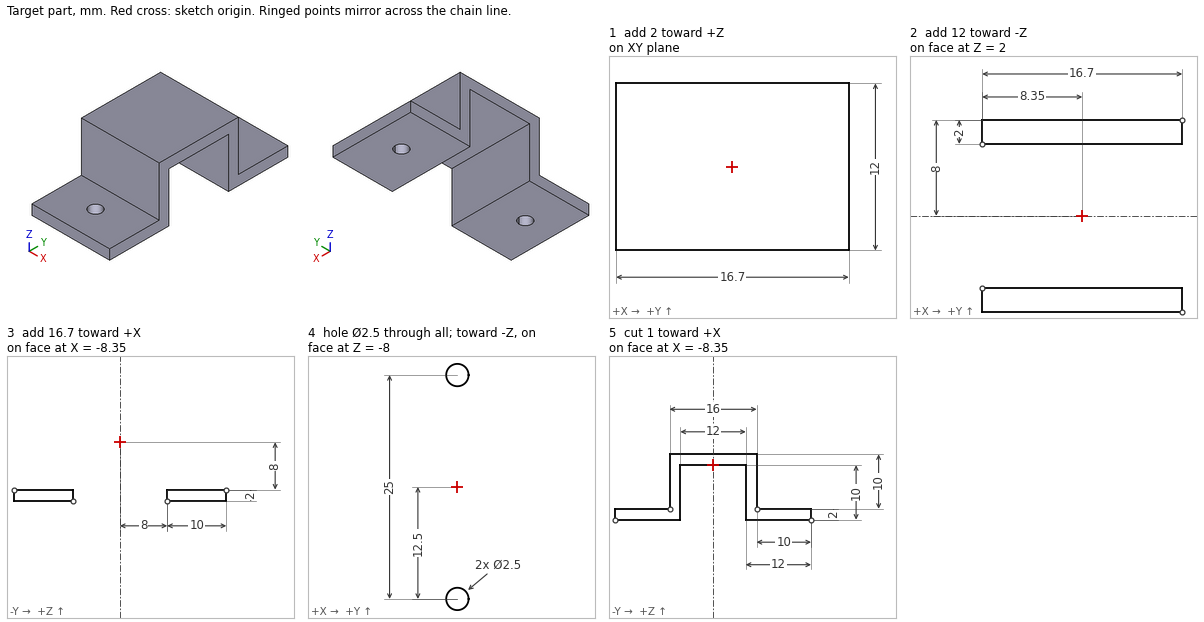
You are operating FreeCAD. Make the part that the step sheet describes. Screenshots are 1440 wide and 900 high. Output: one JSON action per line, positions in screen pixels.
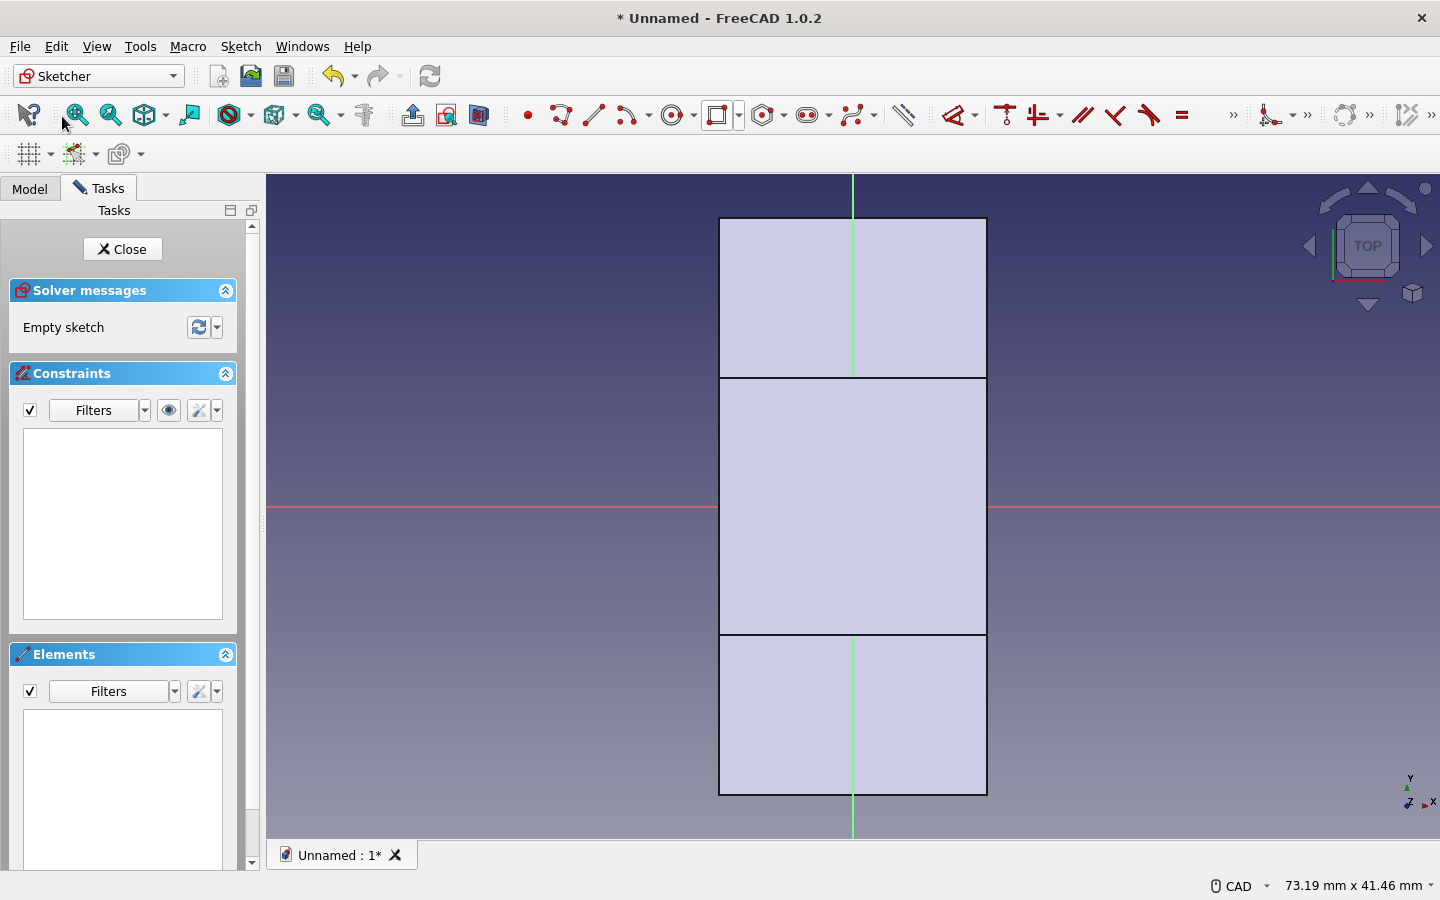
{"action": "left_click", "coordinate": [479, 116]}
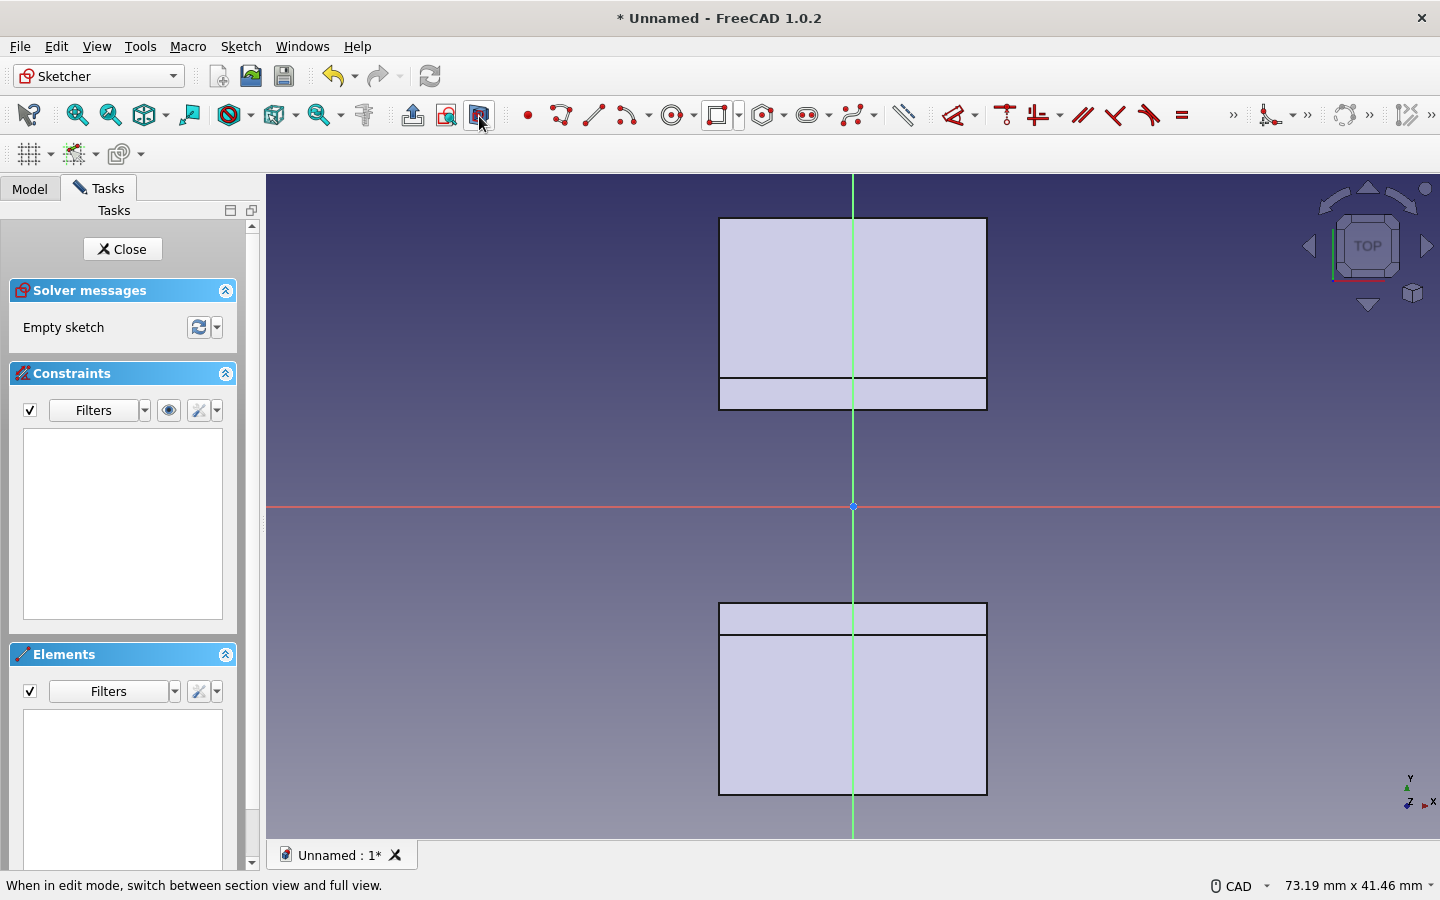
{"action": "left_click", "coordinate": [672, 116]}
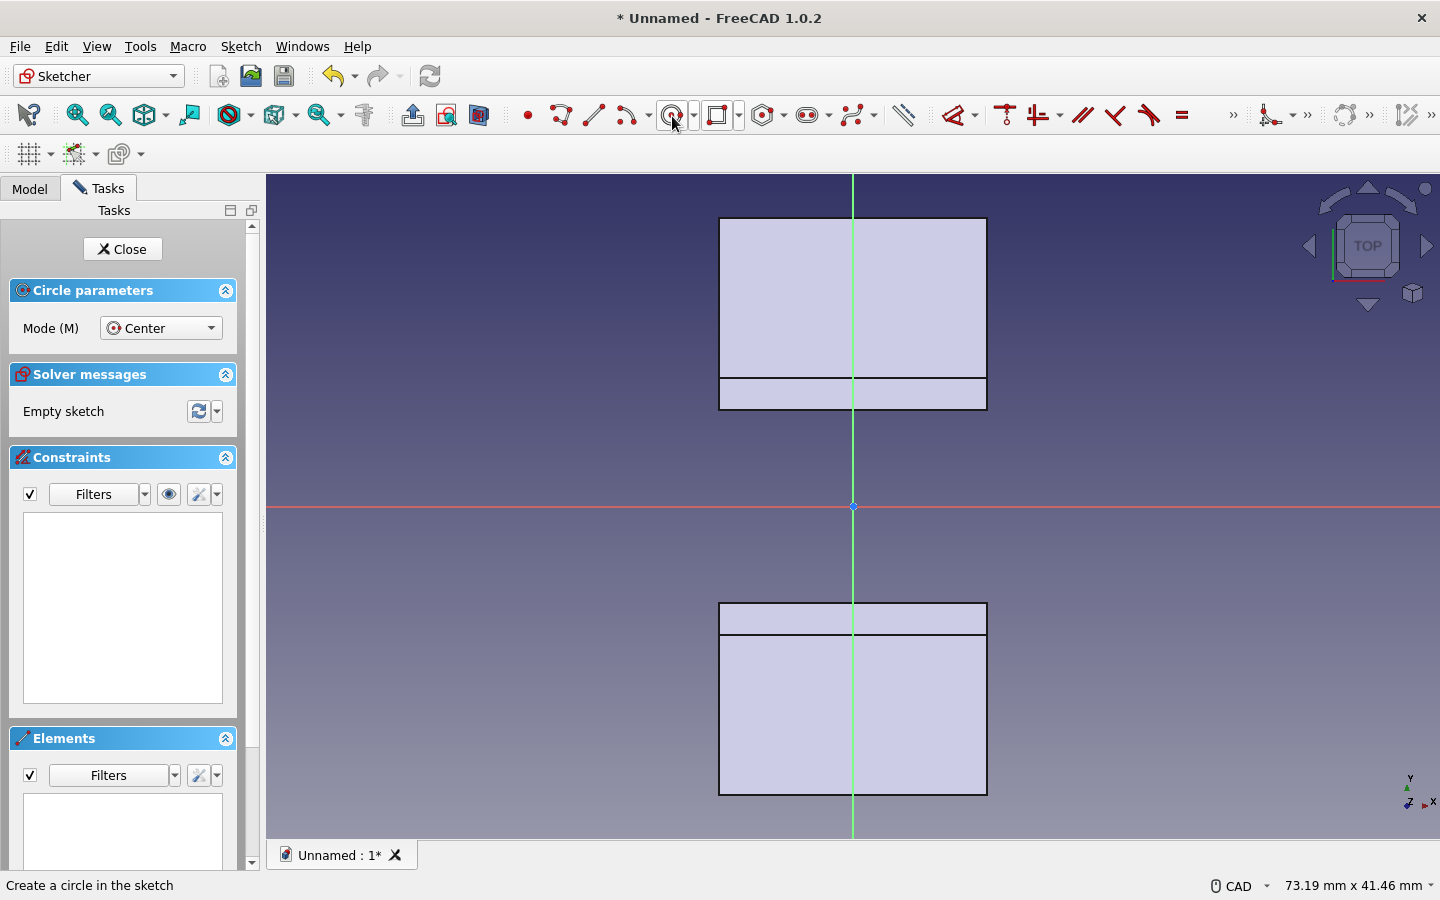
{"action": "left_click", "coordinate": [853, 707]}
{"action": "left_click", "coordinate": [867, 693]}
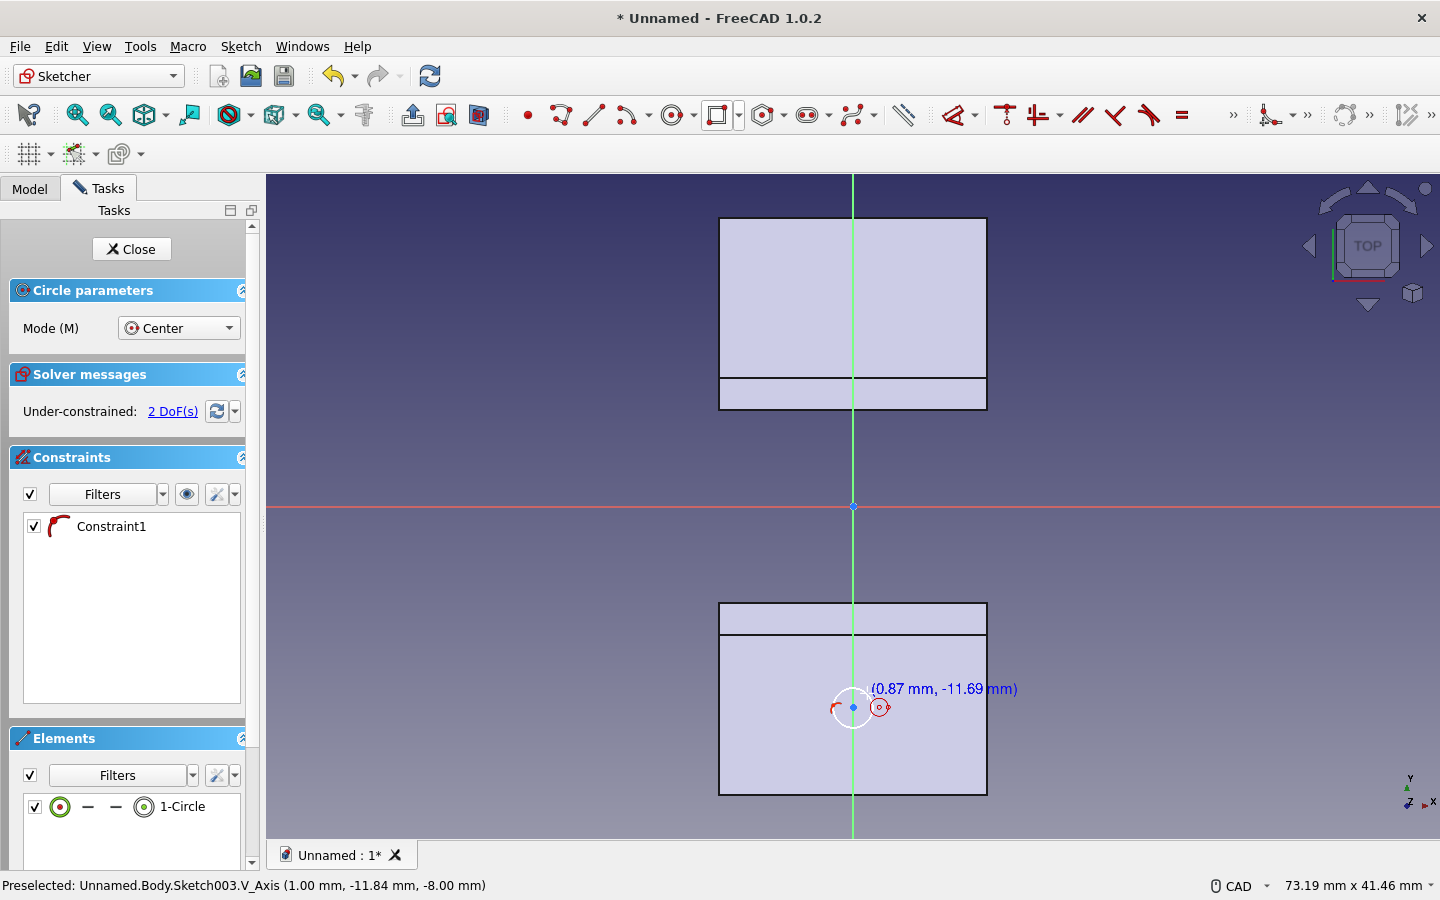
{"action": "left_click", "coordinate": [853, 306]}
{"action": "left_click", "coordinate": [867, 292]}
{"action": "key", "text": "Escape"}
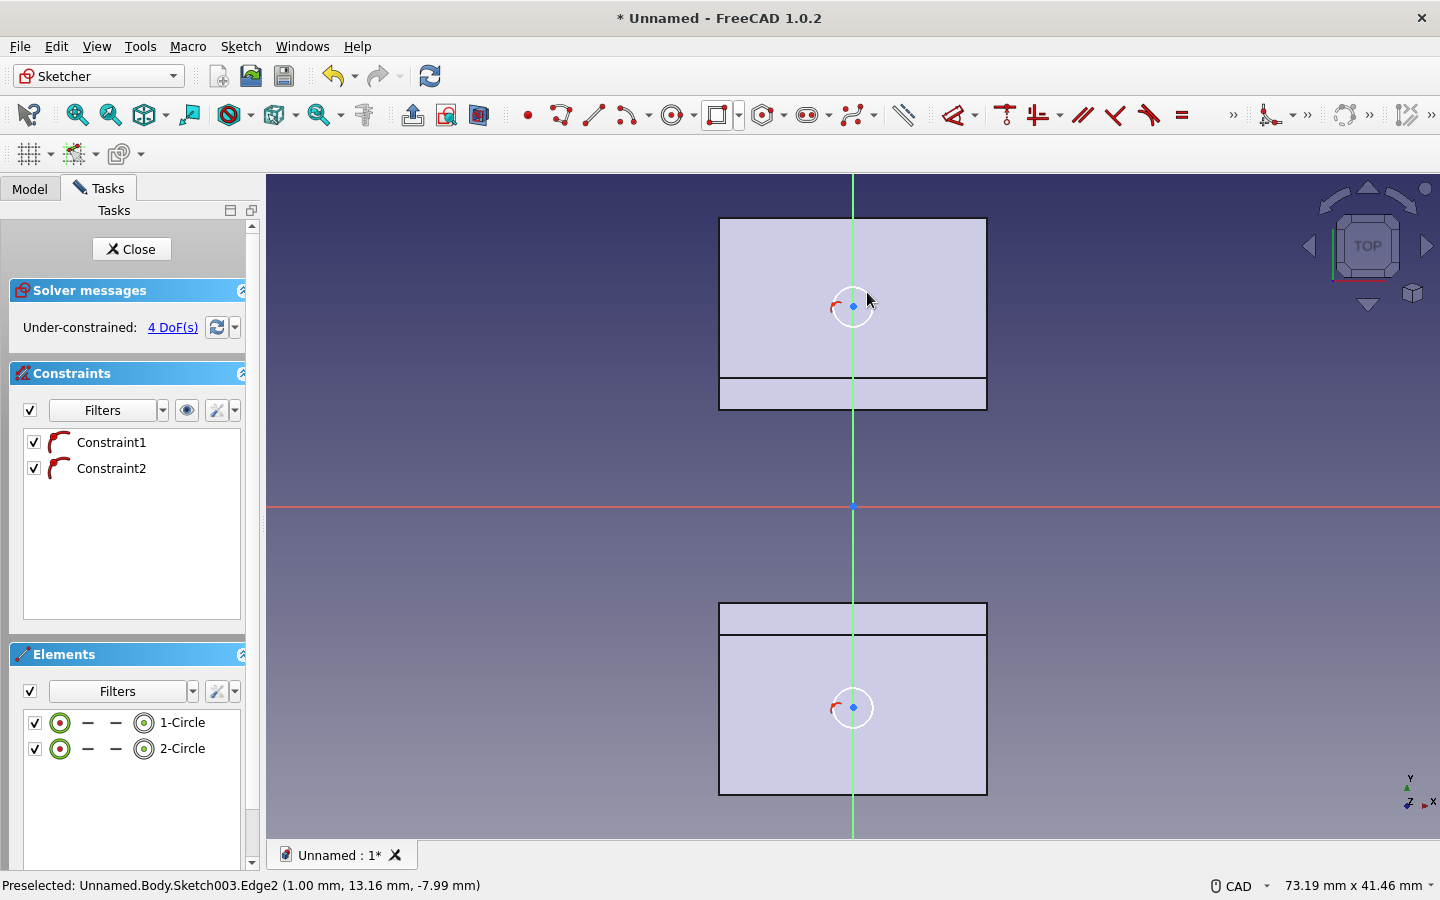
{"action": "left_click", "coordinate": [867, 694]}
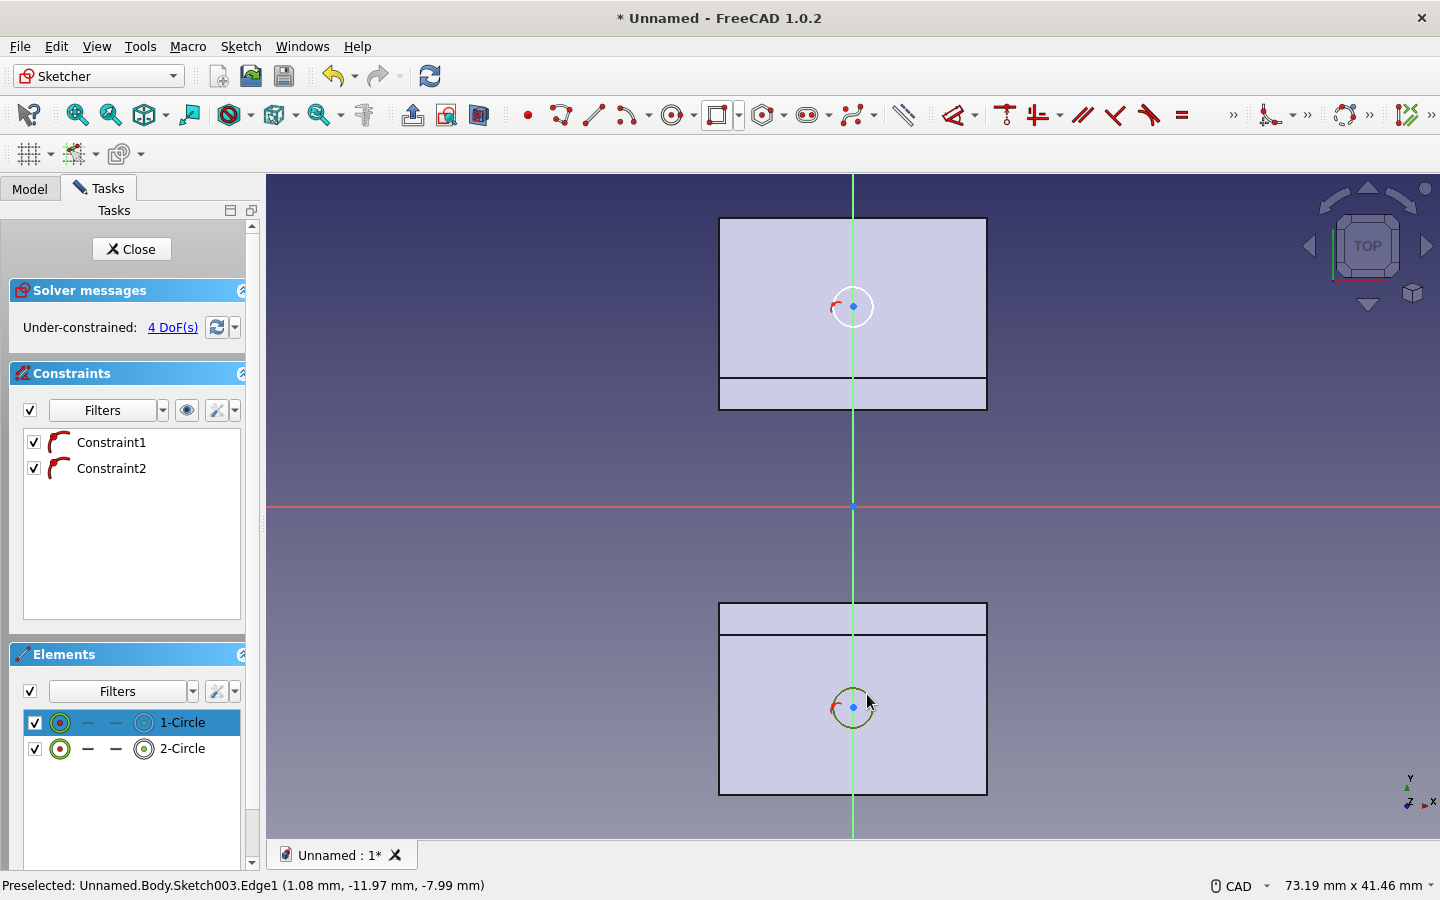
{"action": "left_click", "coordinate": [867, 293]}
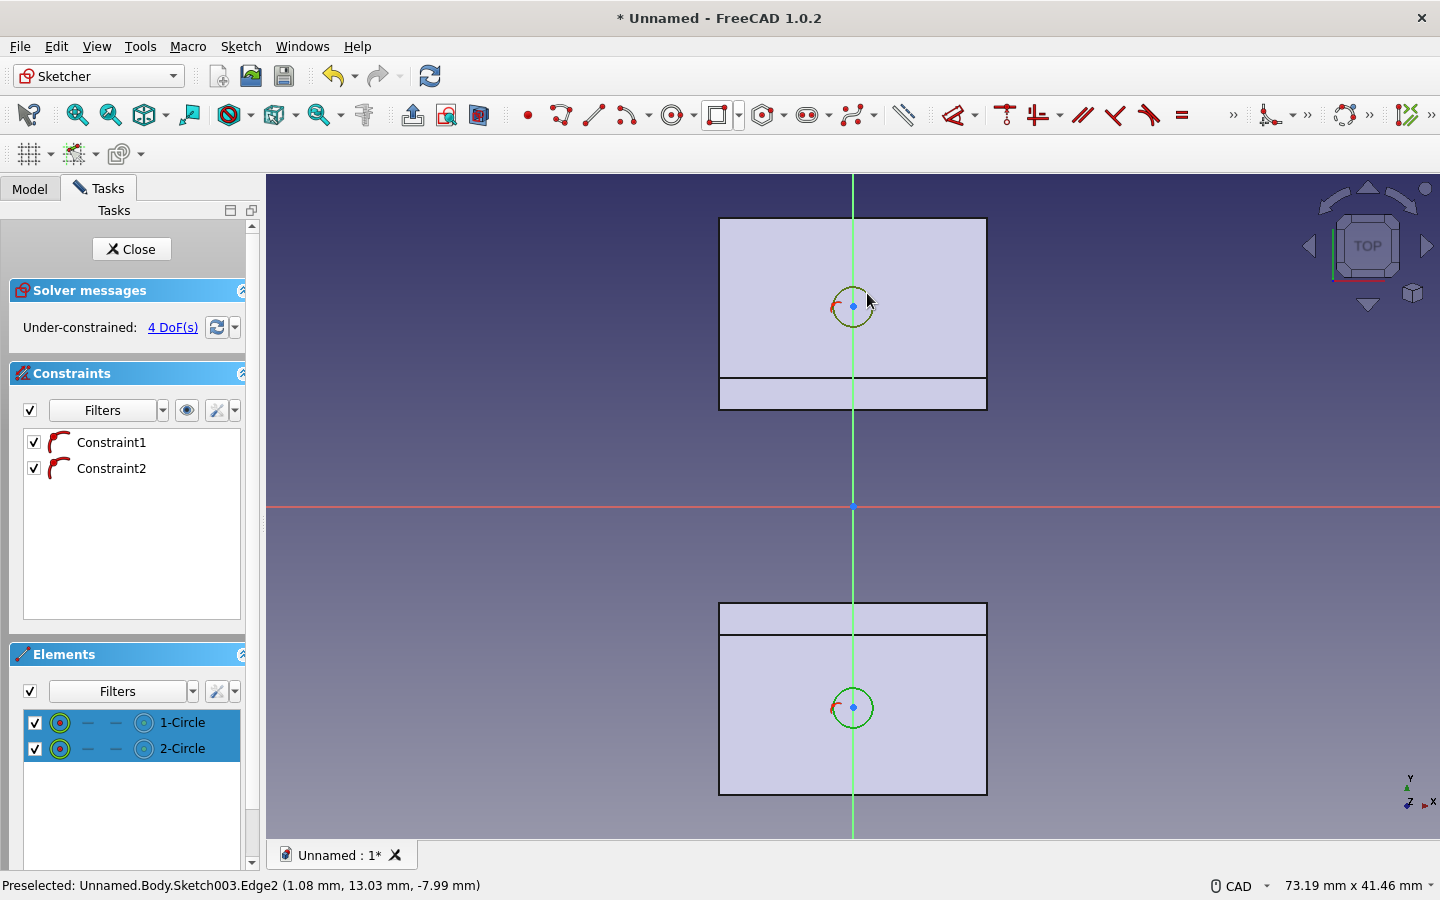
{"action": "key", "text": "e"}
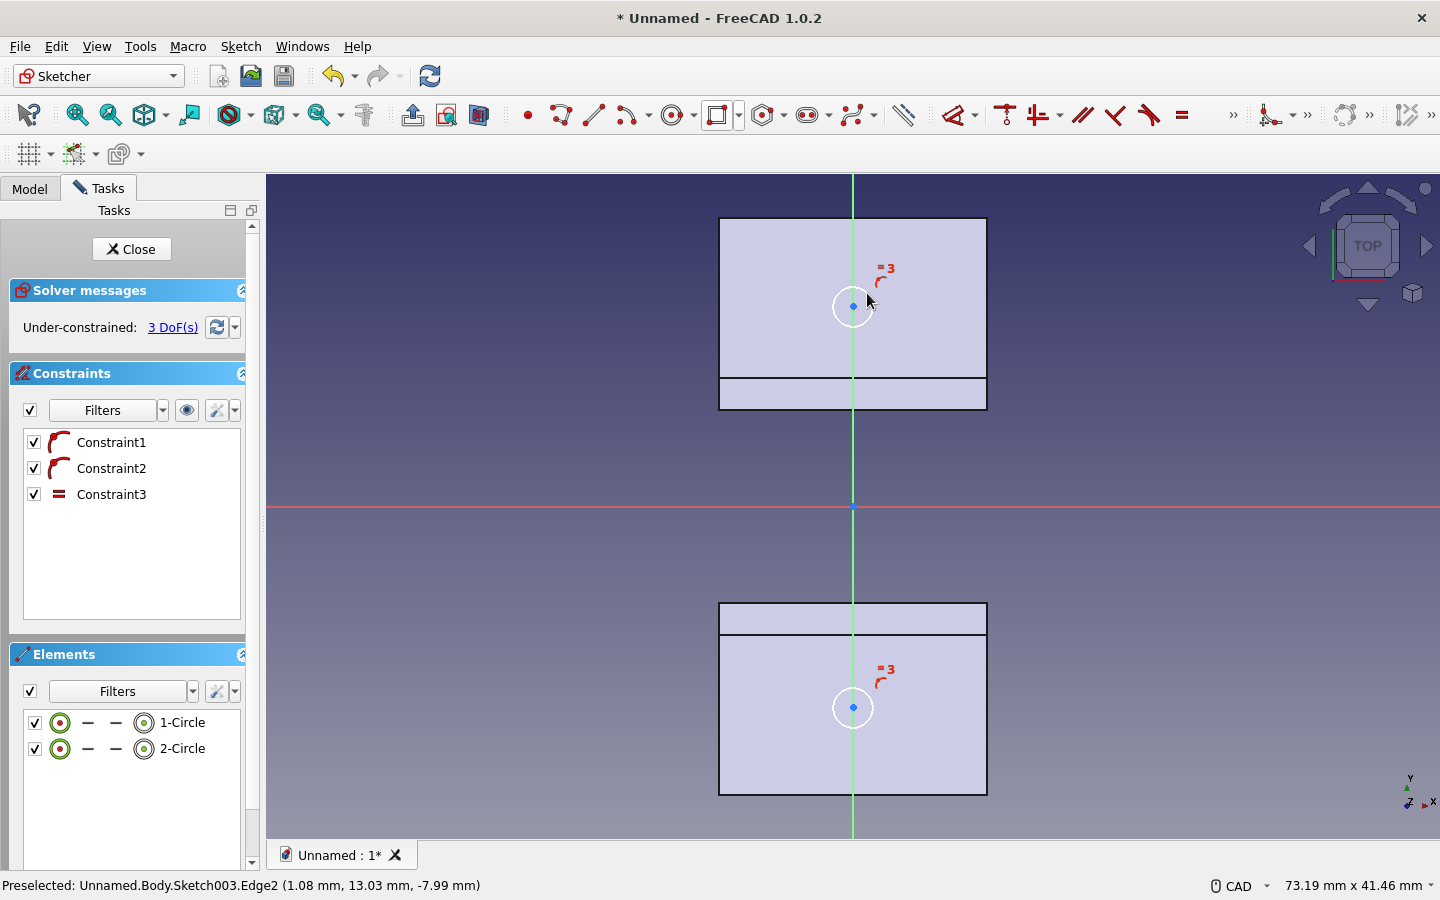
{"action": "left_click", "coordinate": [952, 116]}